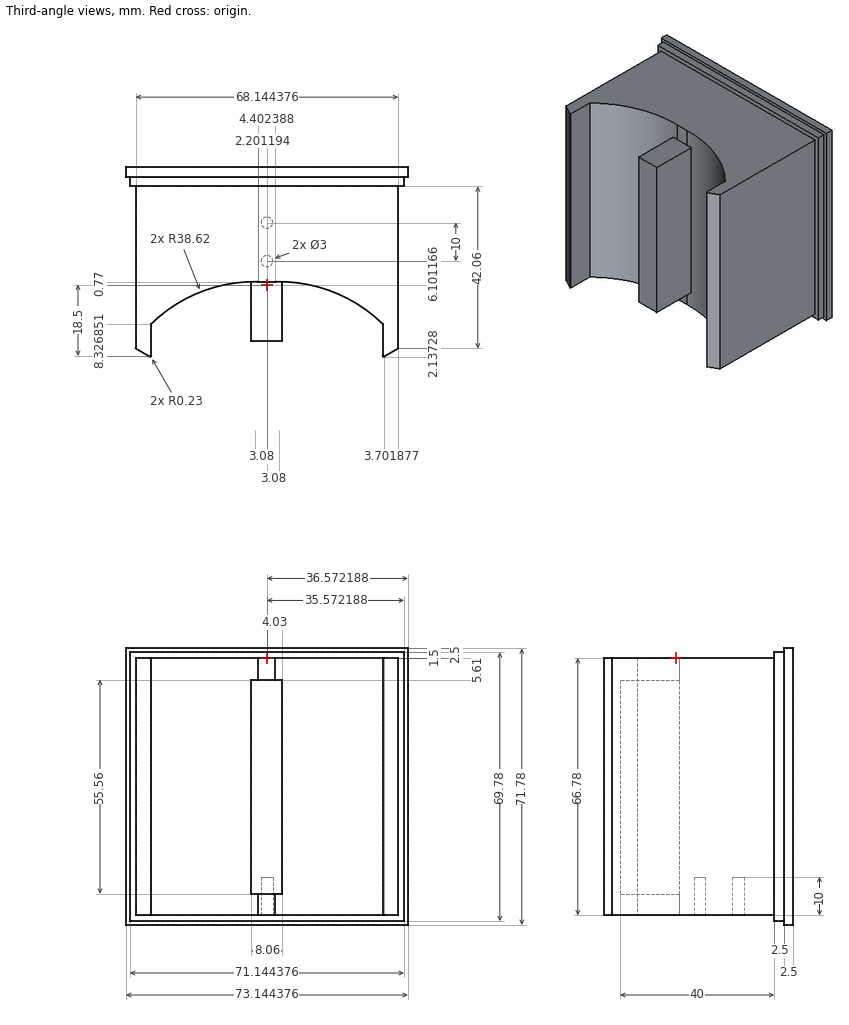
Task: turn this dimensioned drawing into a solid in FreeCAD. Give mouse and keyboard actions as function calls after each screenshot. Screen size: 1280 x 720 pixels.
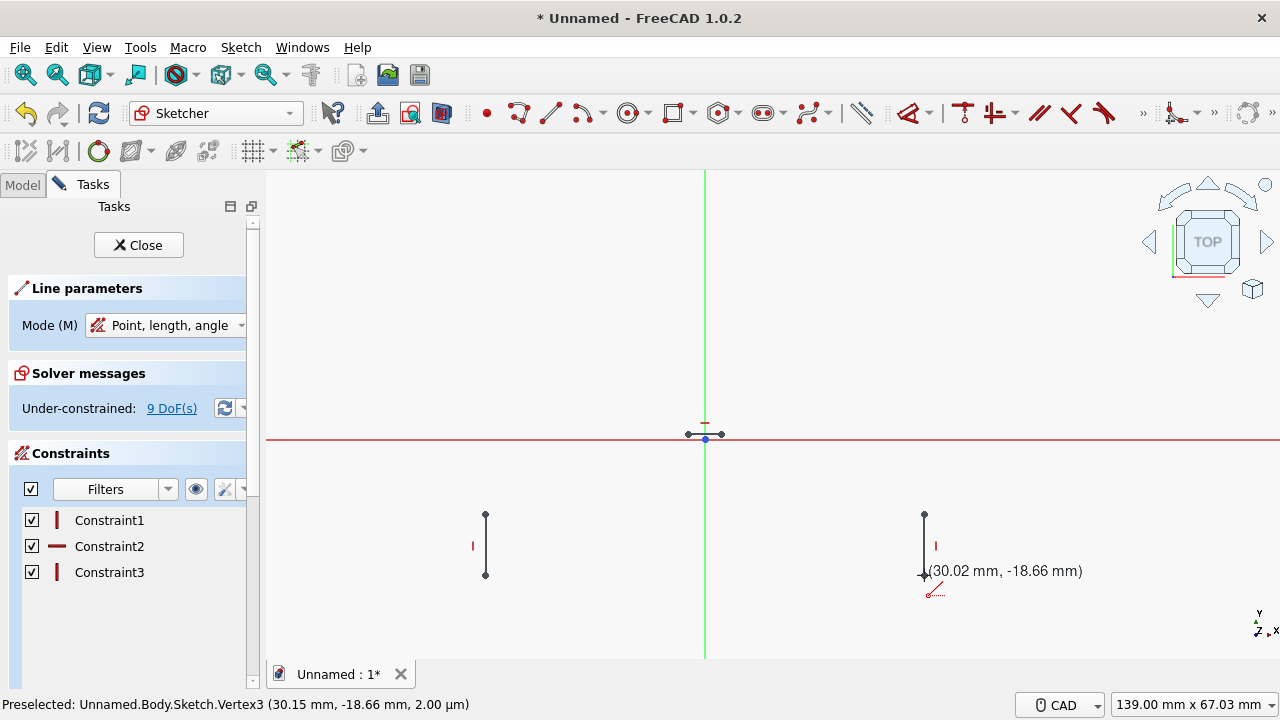
click(520, 114)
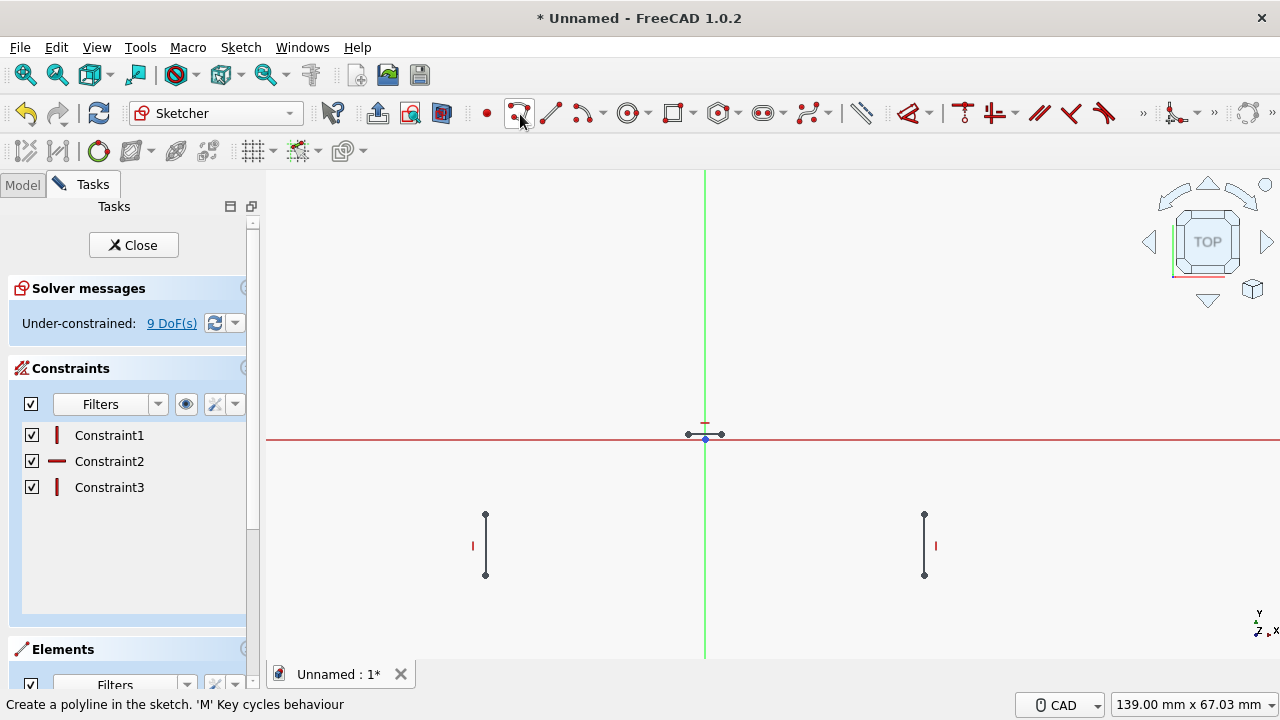
scroll(927, 576, up, 9)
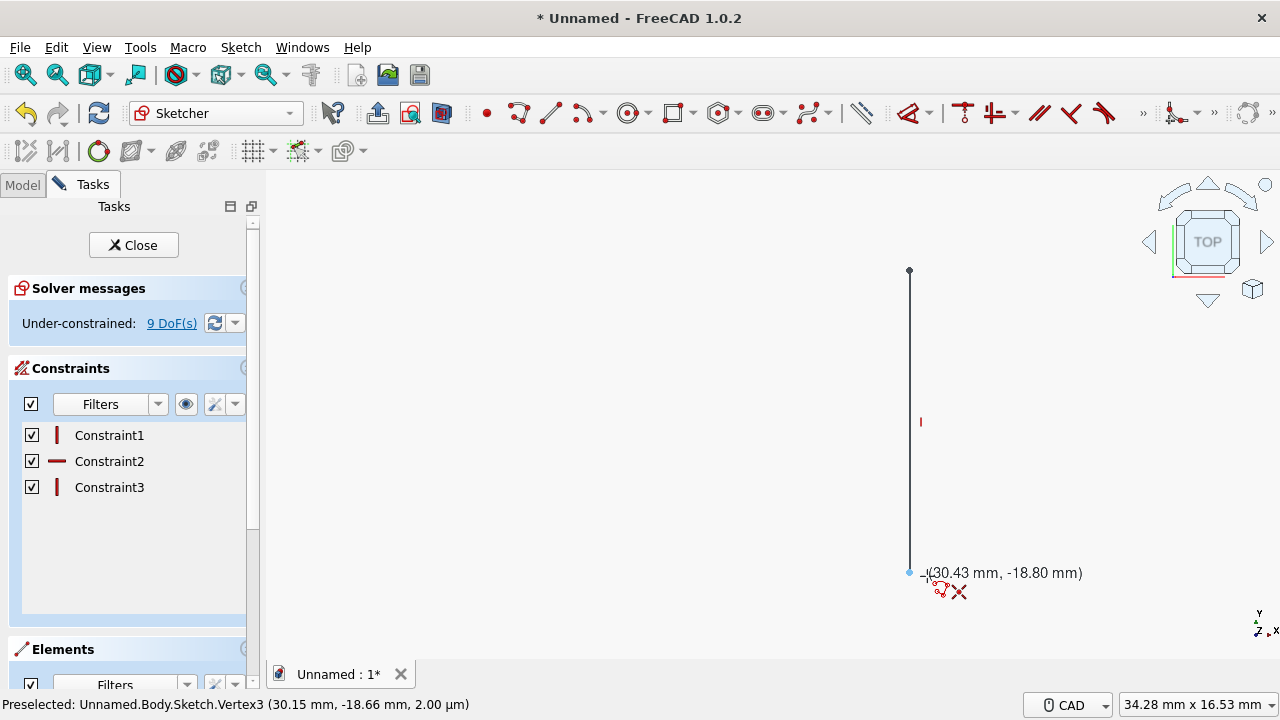
click(921, 573)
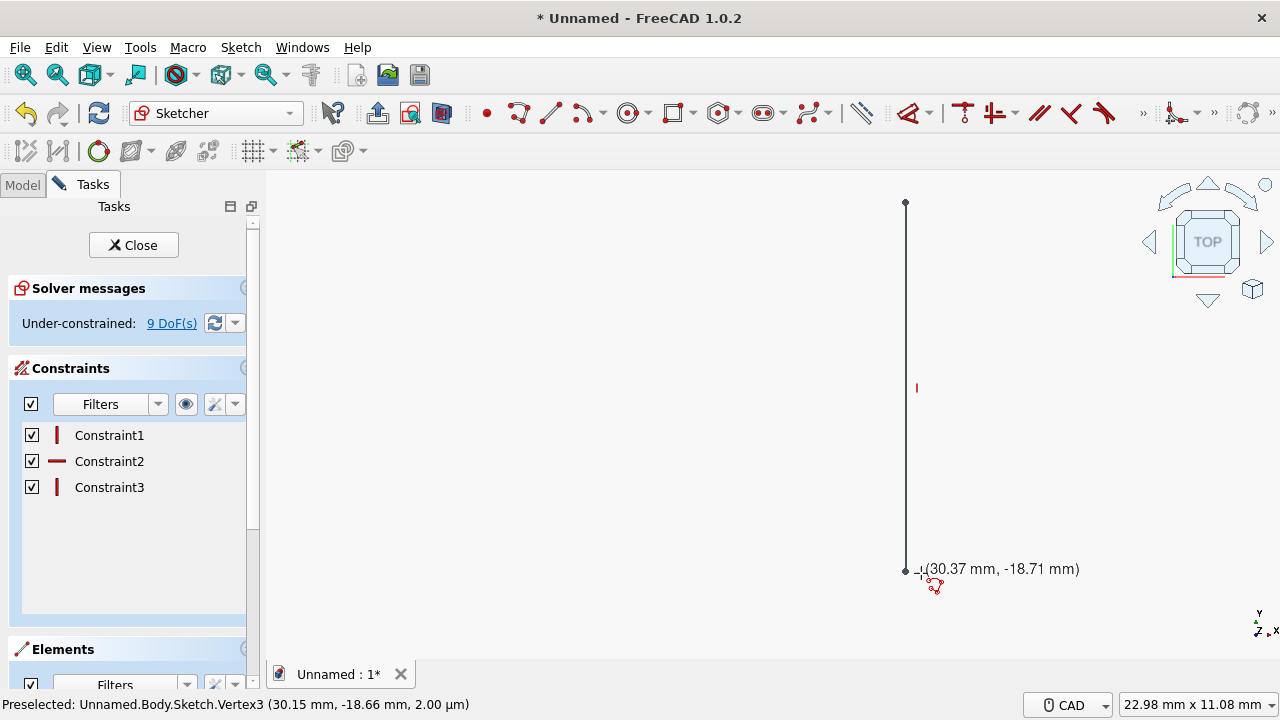
scroll(927, 576, down, 9)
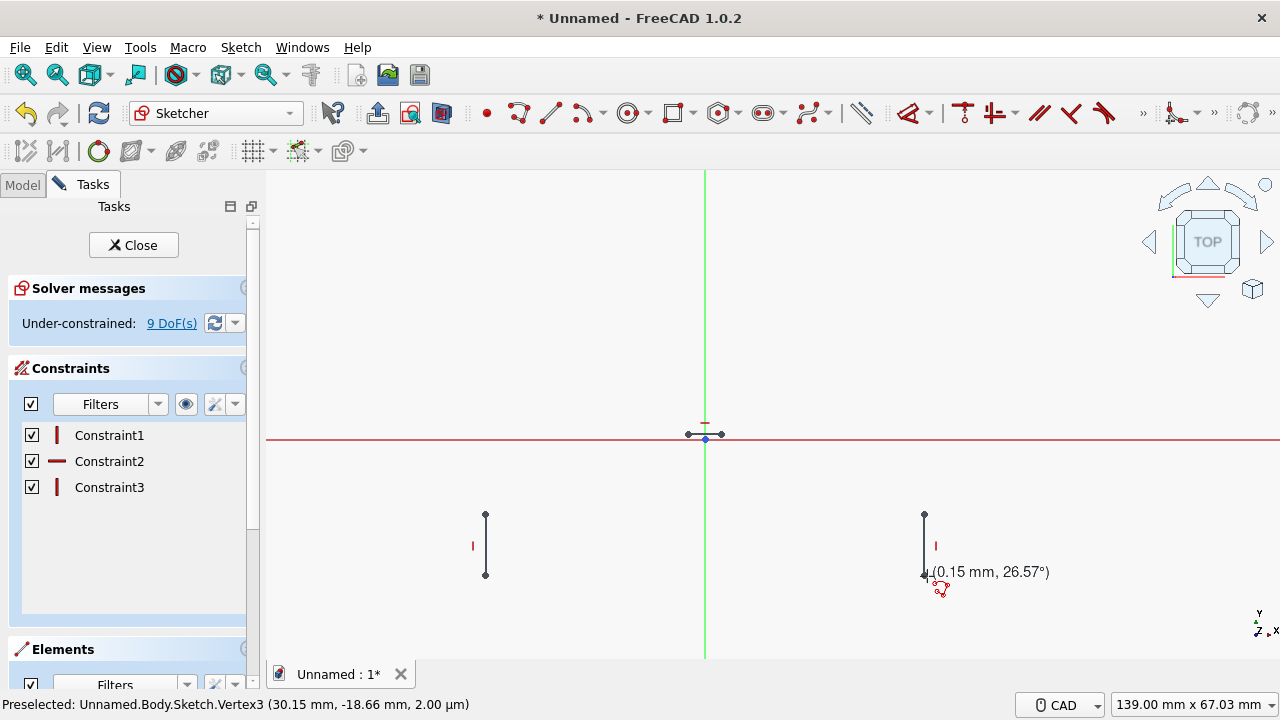
click(954, 561)
click(954, 254)
click(456, 254)
click(456, 561)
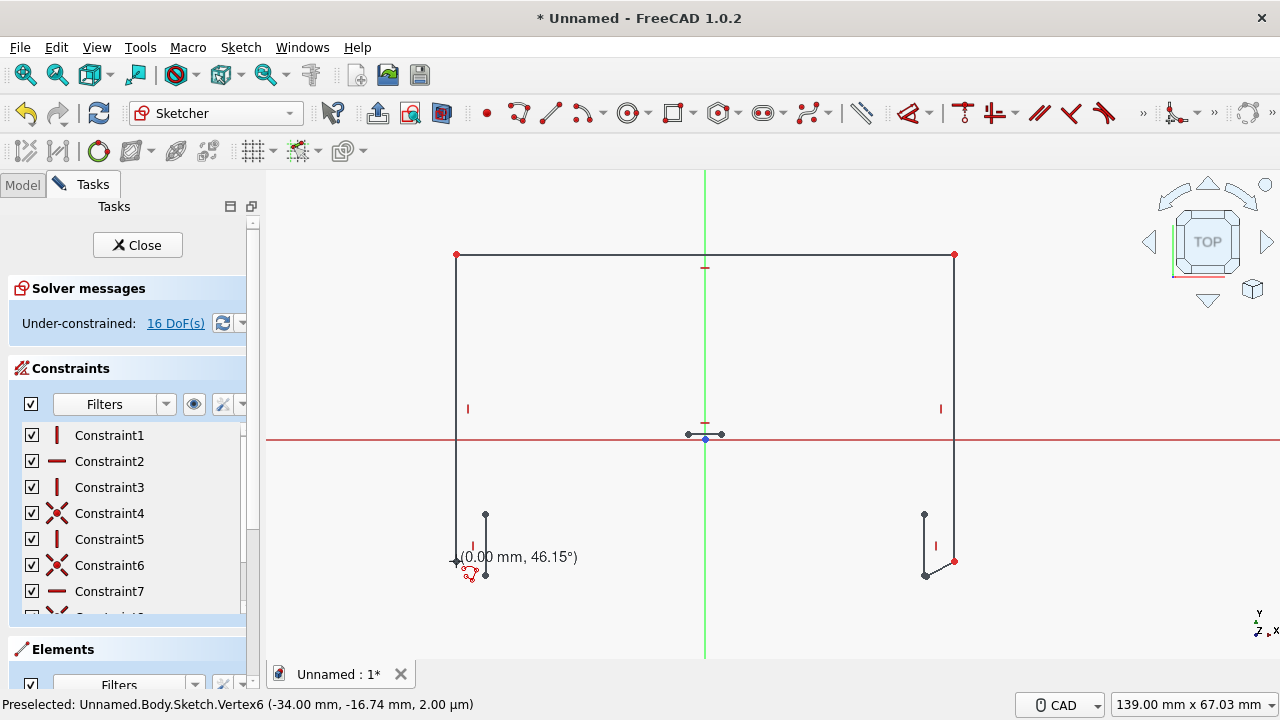
scroll(483, 576, up, 9)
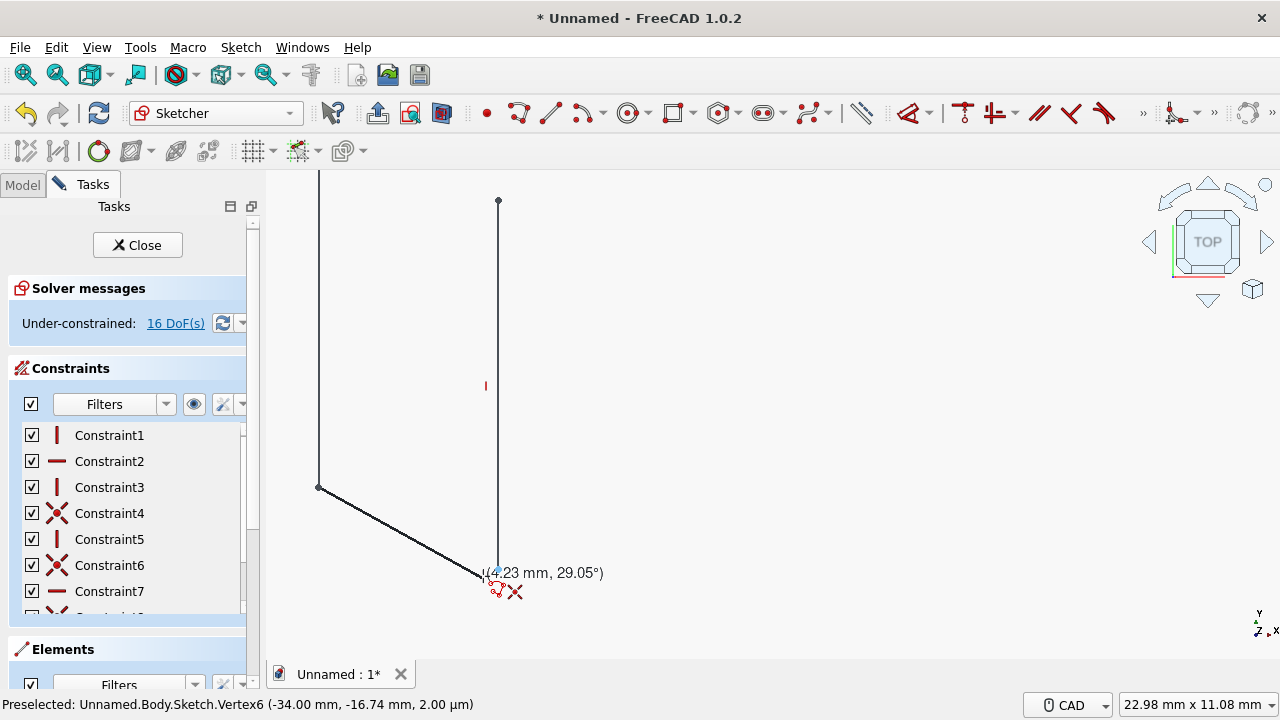
click(485, 573)
right_click(485, 573)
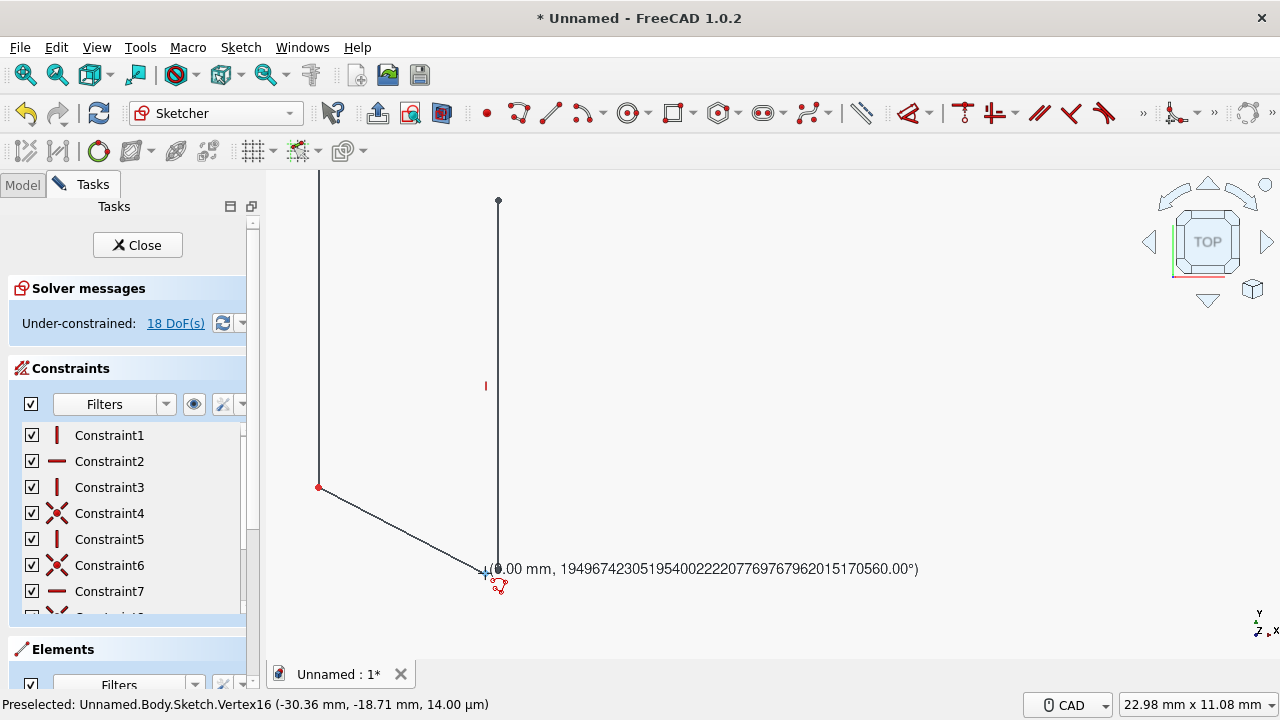
click(606, 114)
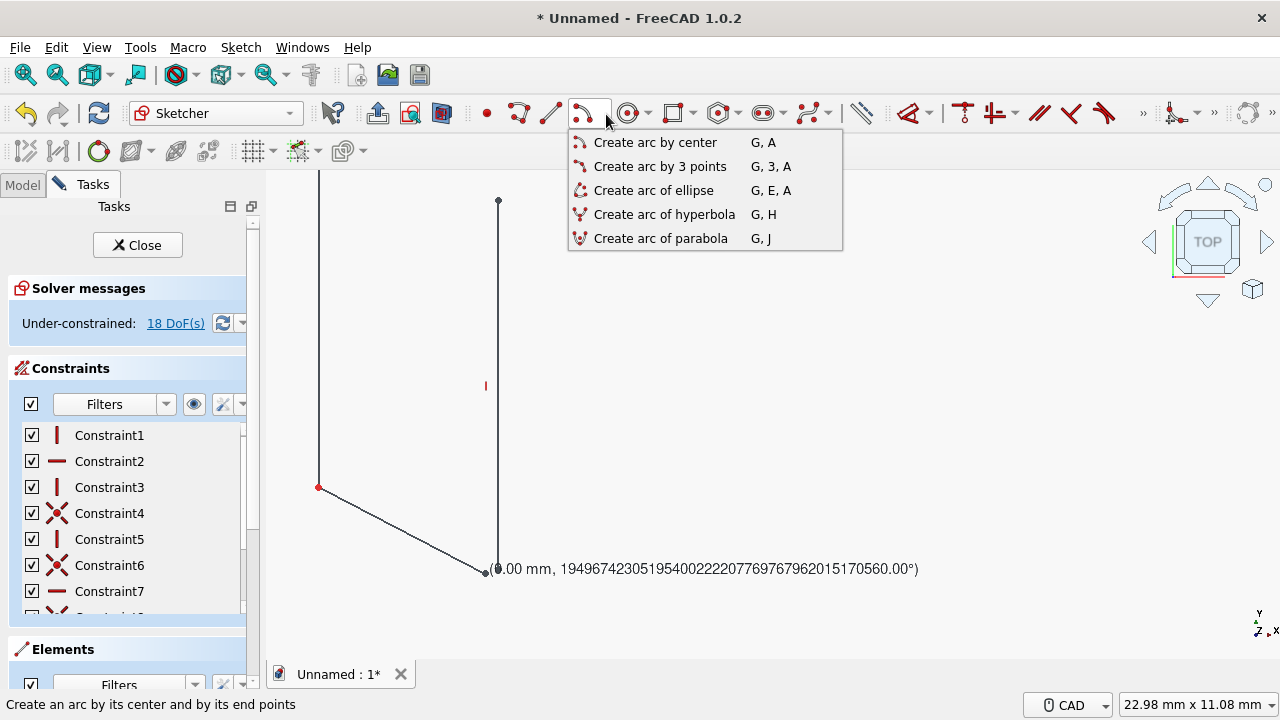
click(706, 166)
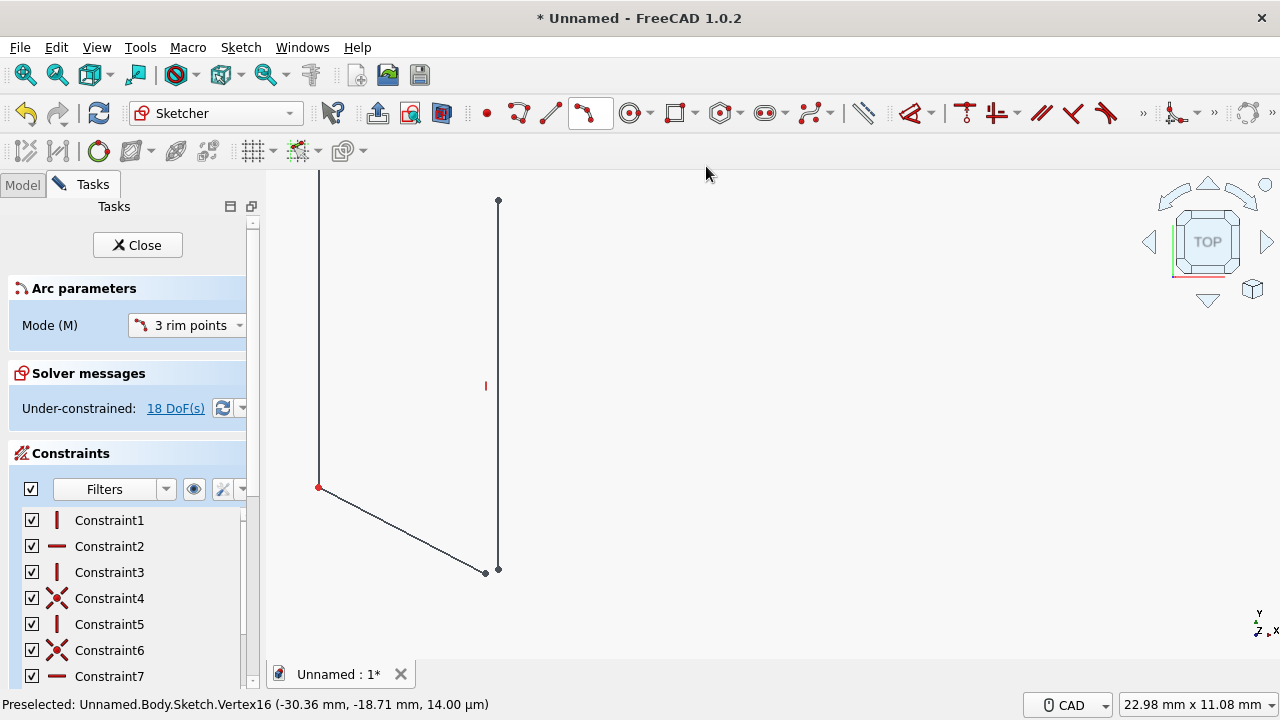
scroll(483, 576, down, 9)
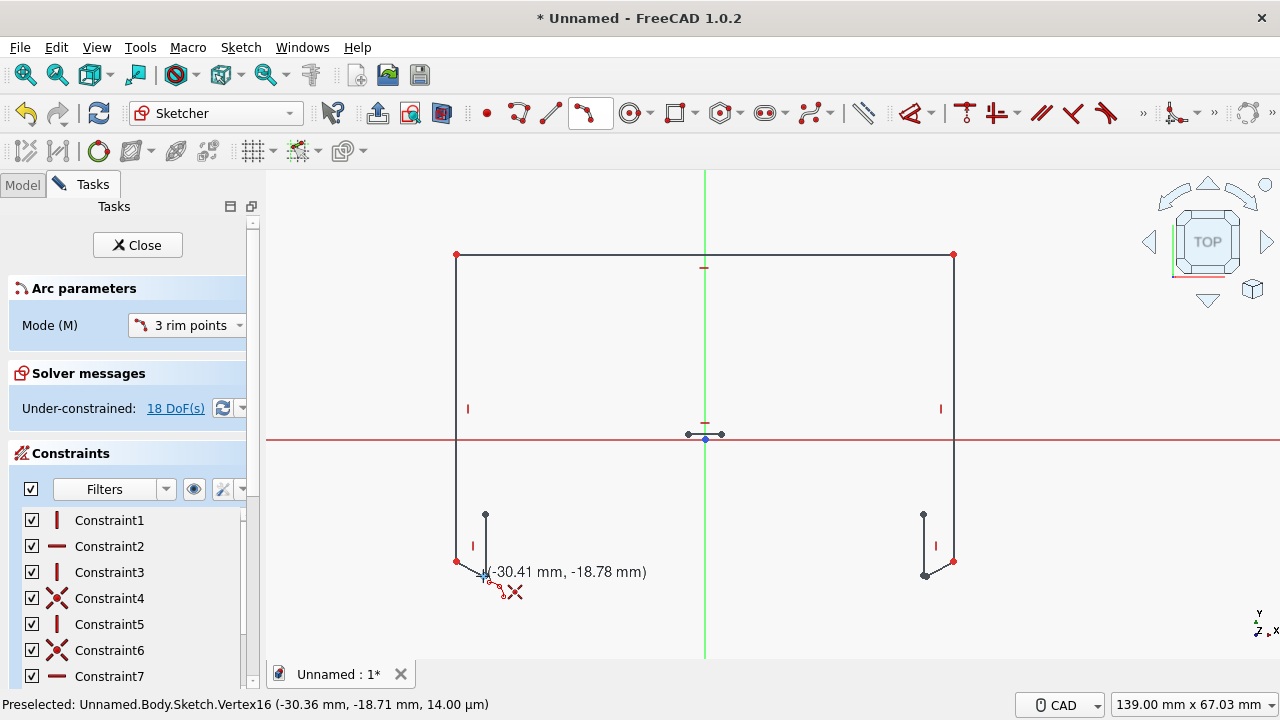
click(486, 515)